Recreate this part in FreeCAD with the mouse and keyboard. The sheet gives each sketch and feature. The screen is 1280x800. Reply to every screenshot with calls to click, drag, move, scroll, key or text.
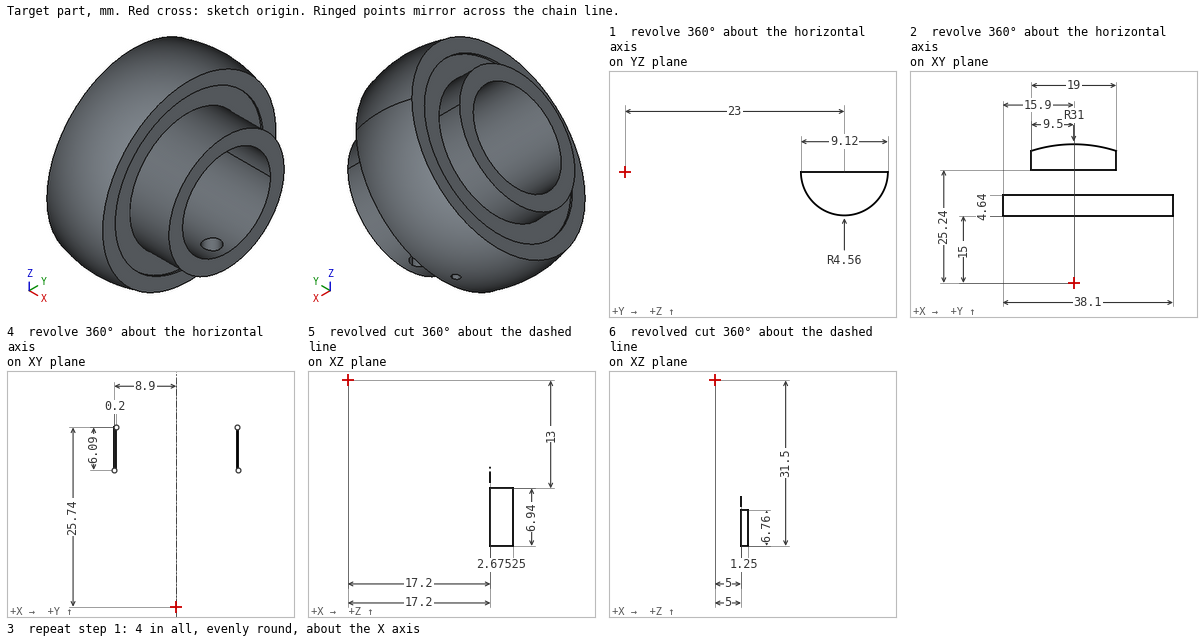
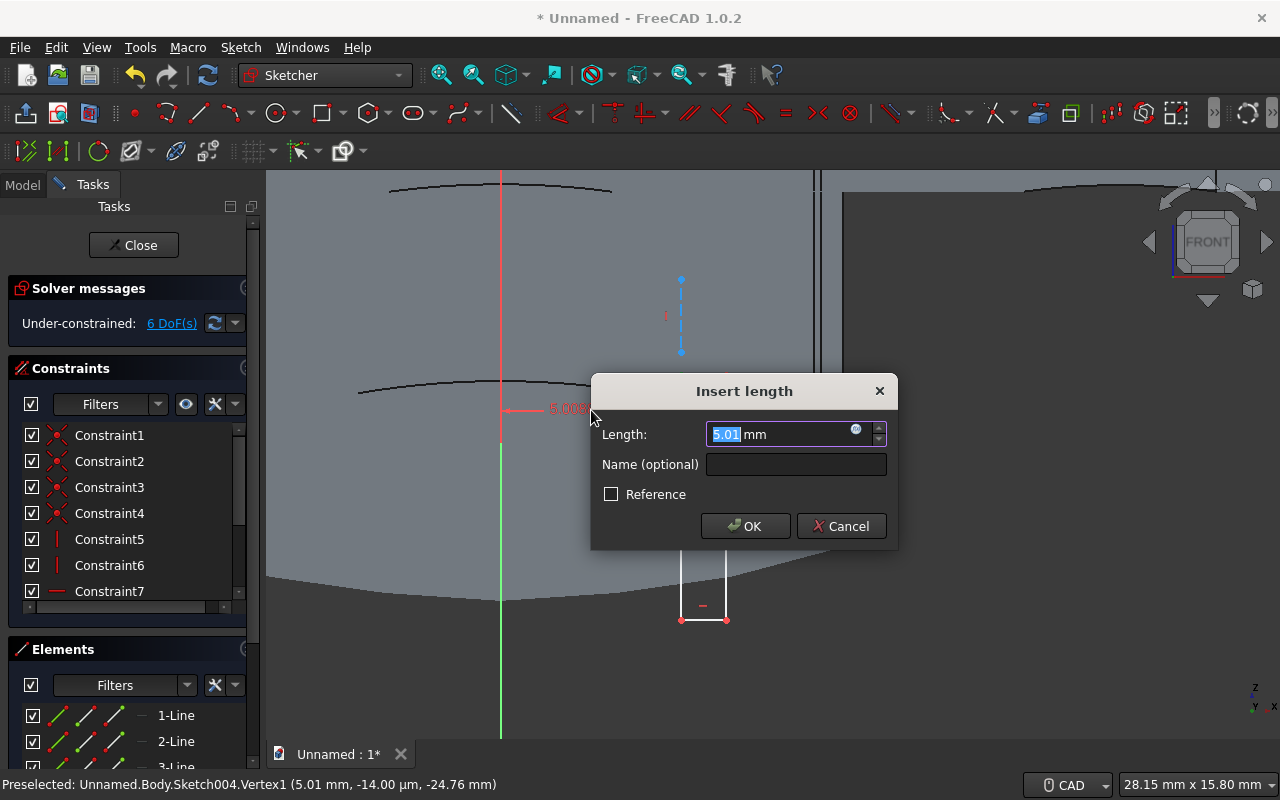
text(5)
key(Return)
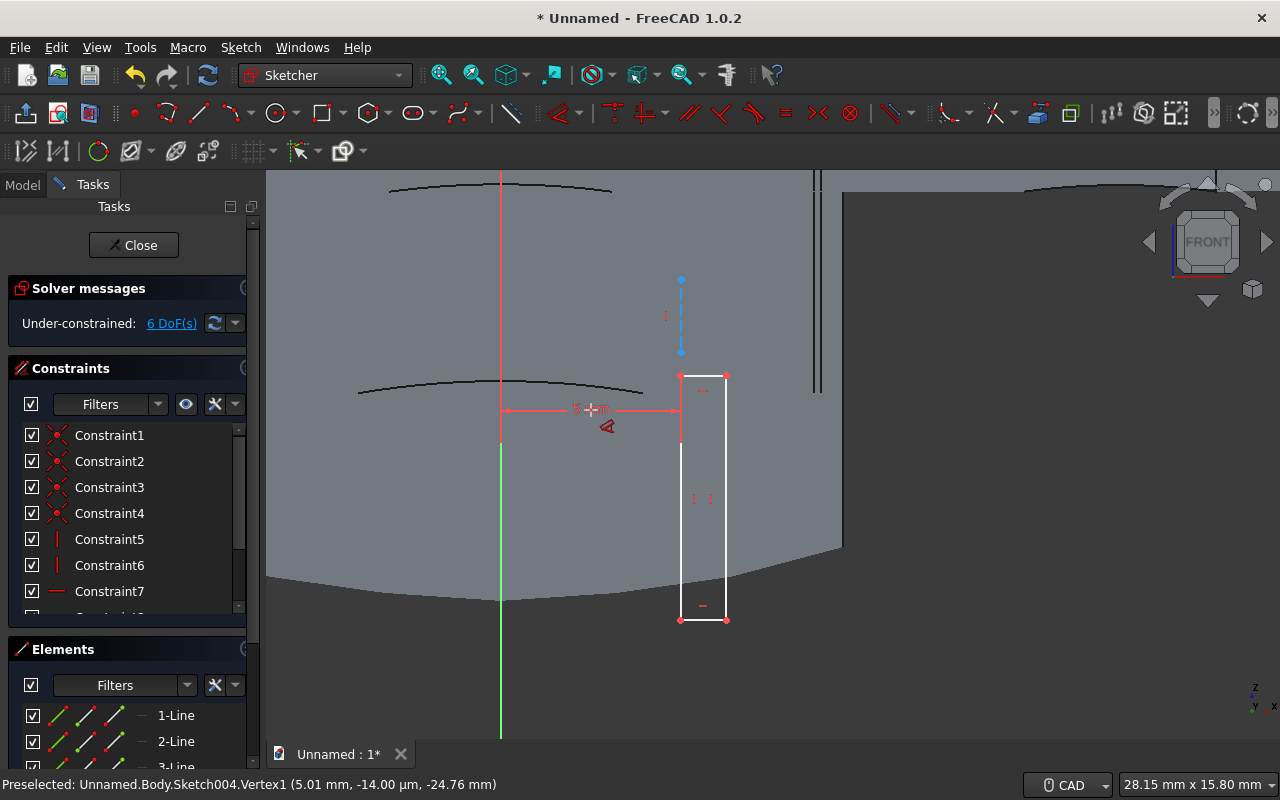
click(681, 352)
click(591, 386)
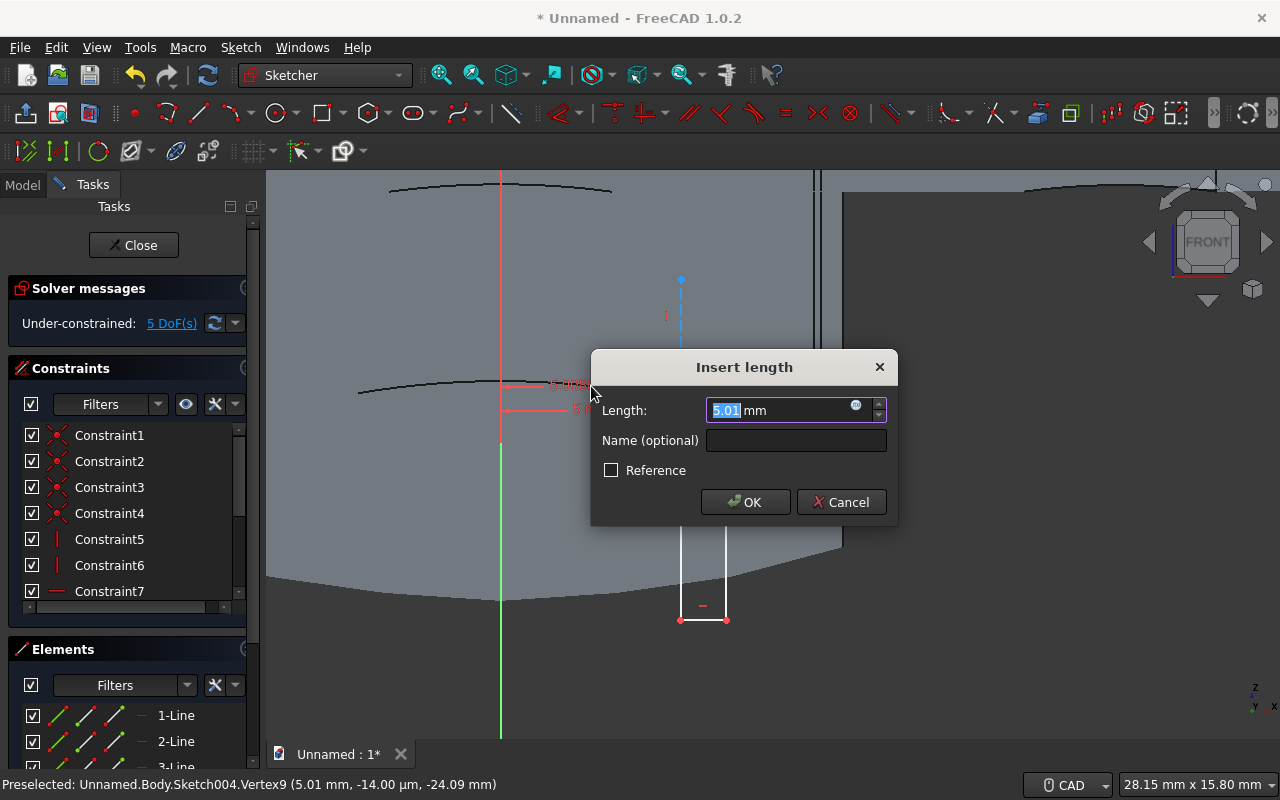
text(5)
key(Return)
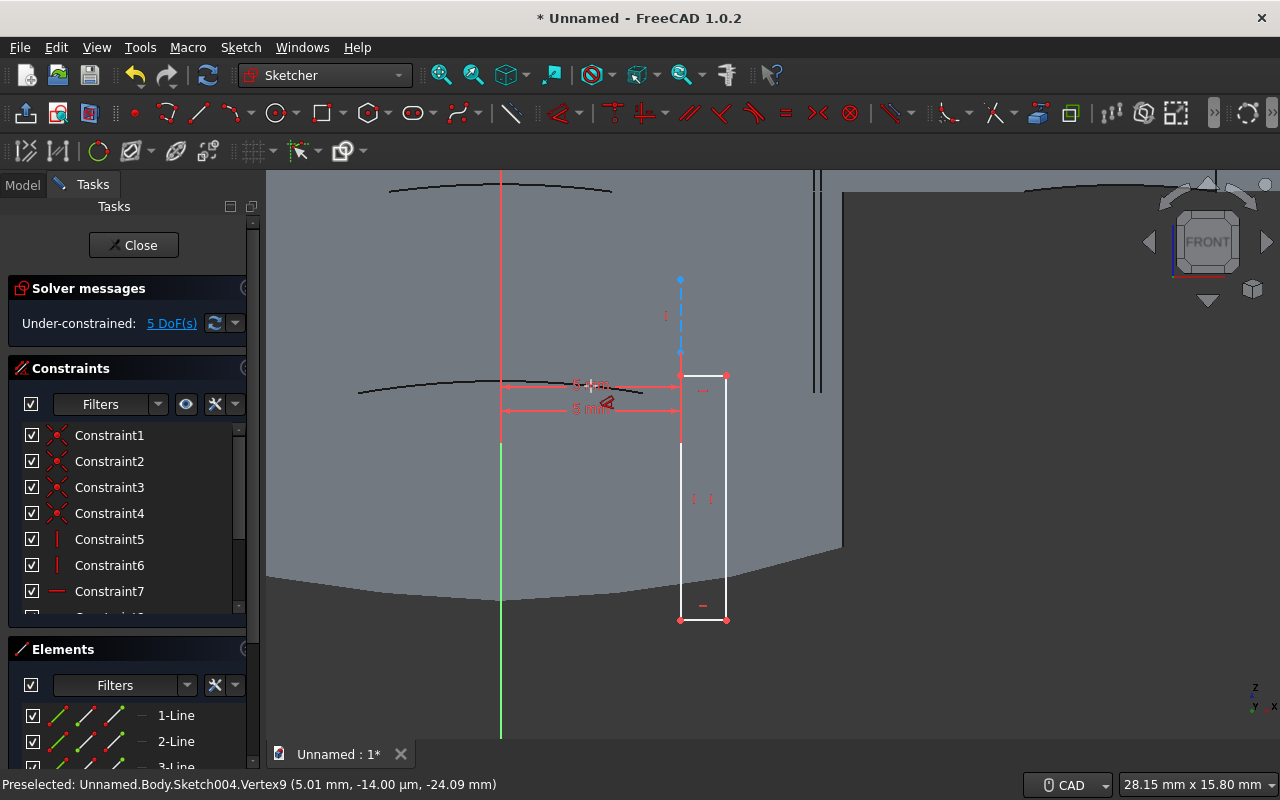
click(681, 449)
click(647, 498)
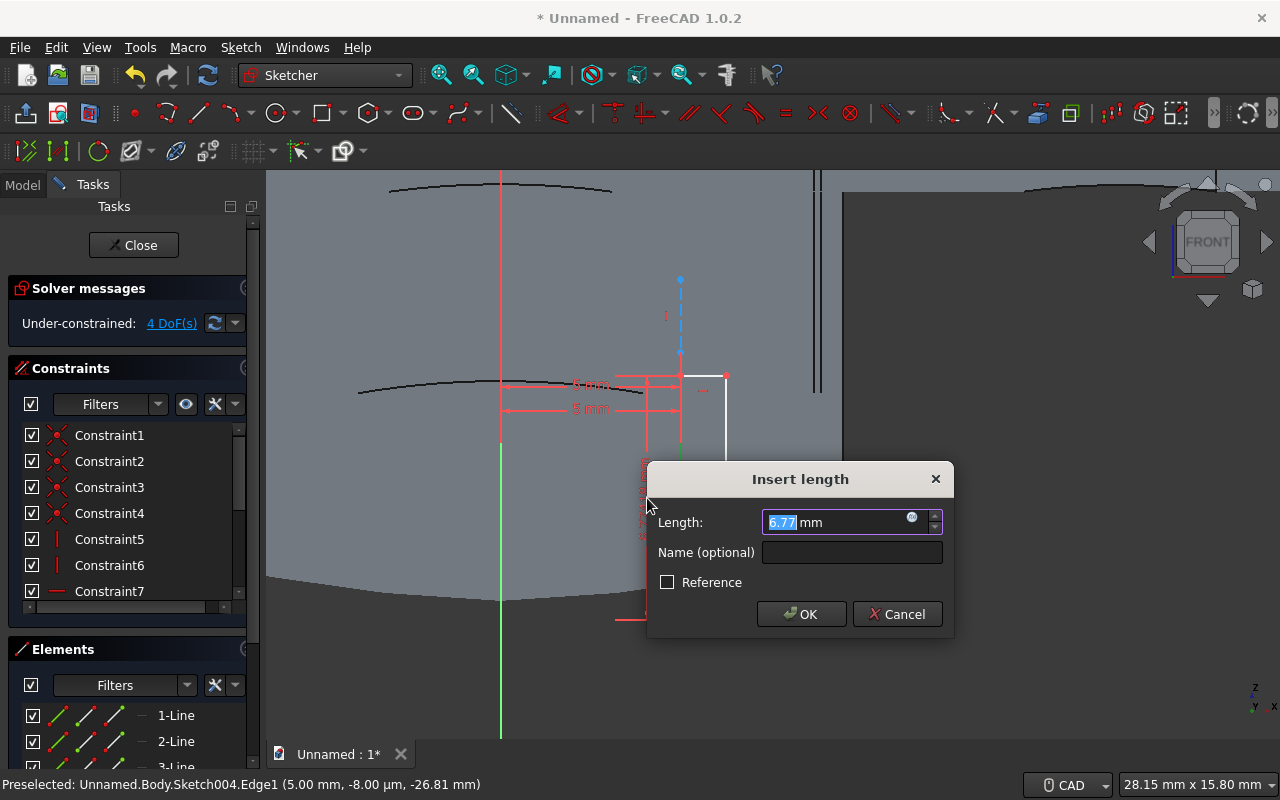
text(6.76)
key(Return)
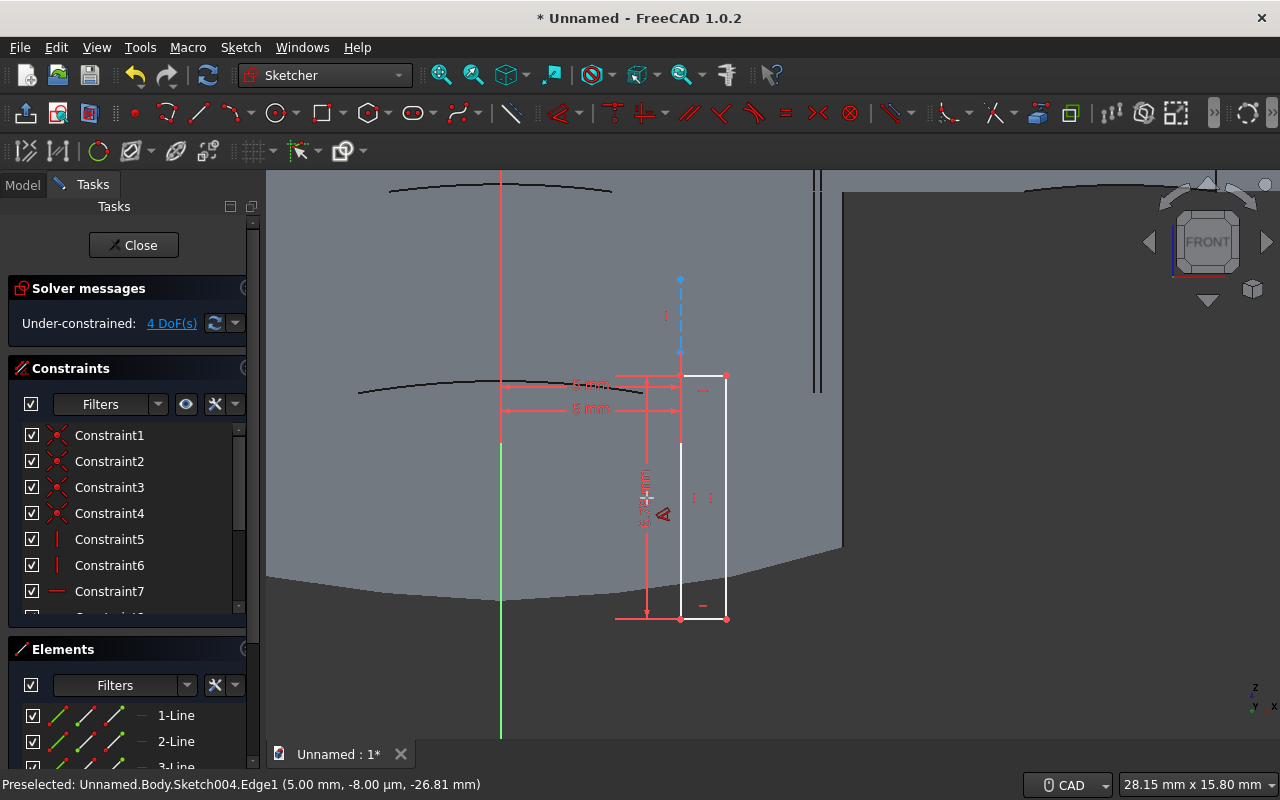
click(694, 619)
click(703, 653)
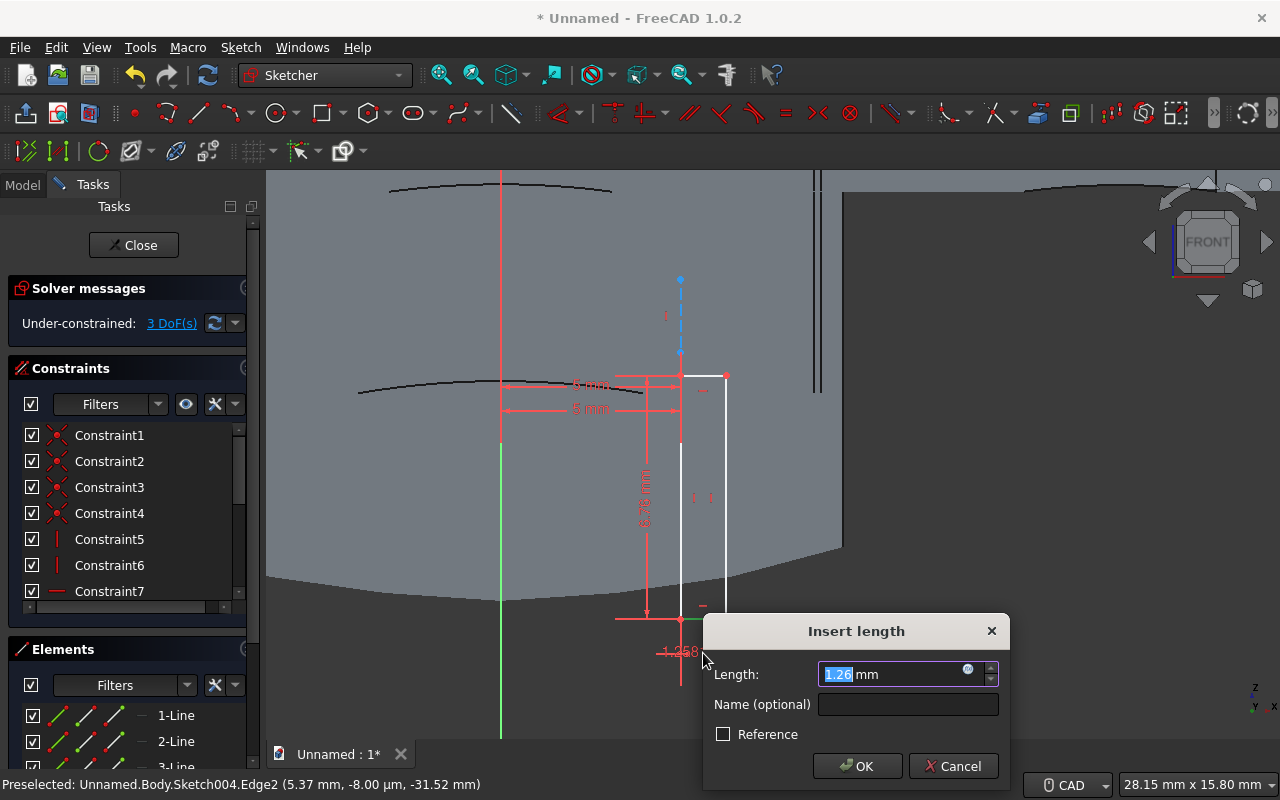
text(1.25)
key(Return)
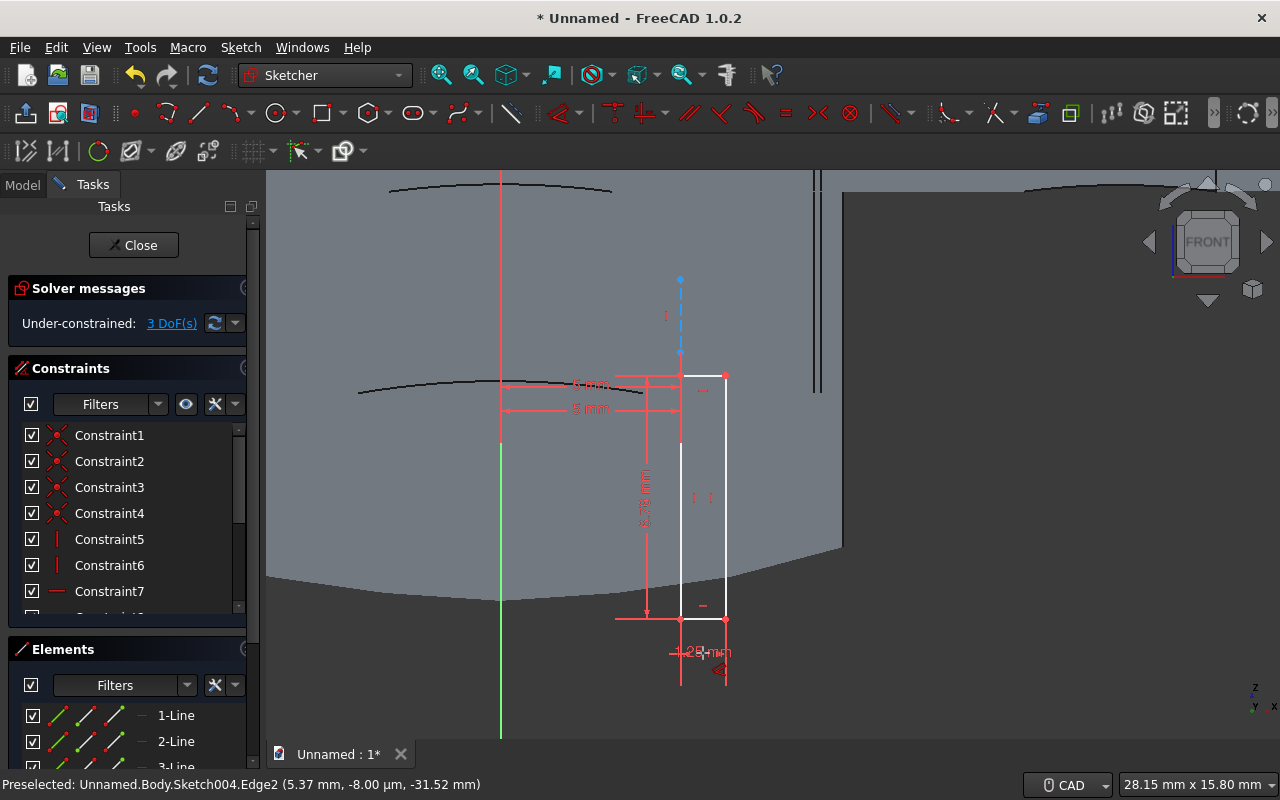
click(681, 619)
click(467, 409)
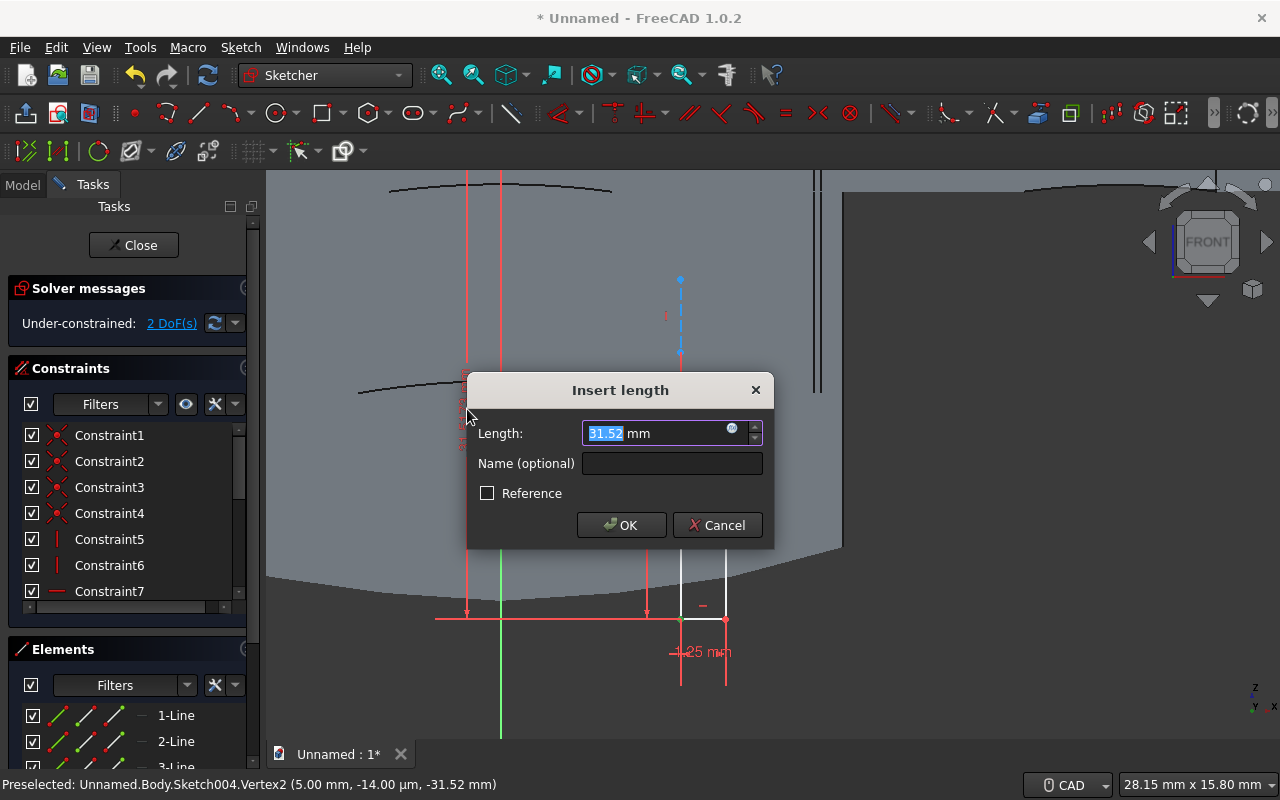
text(31.5)
key(Return)
key(Escape)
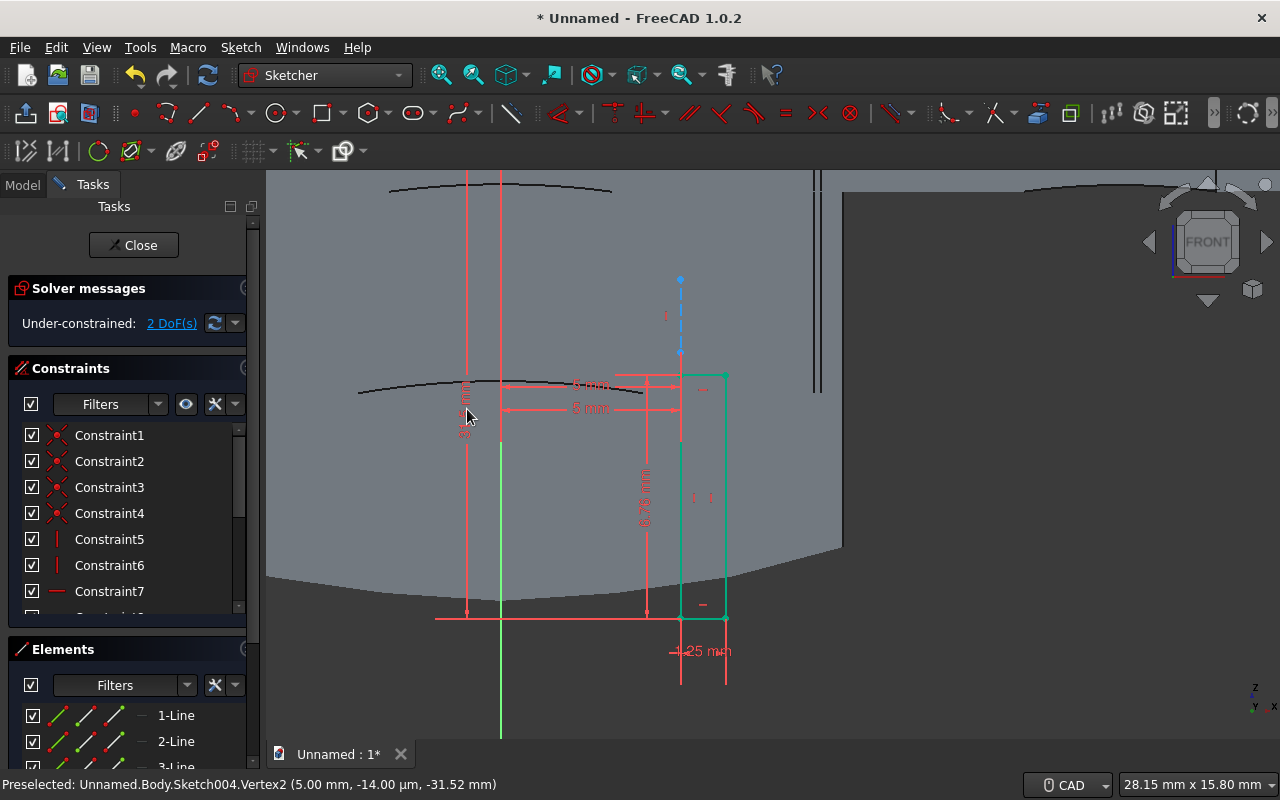
click(134, 245)